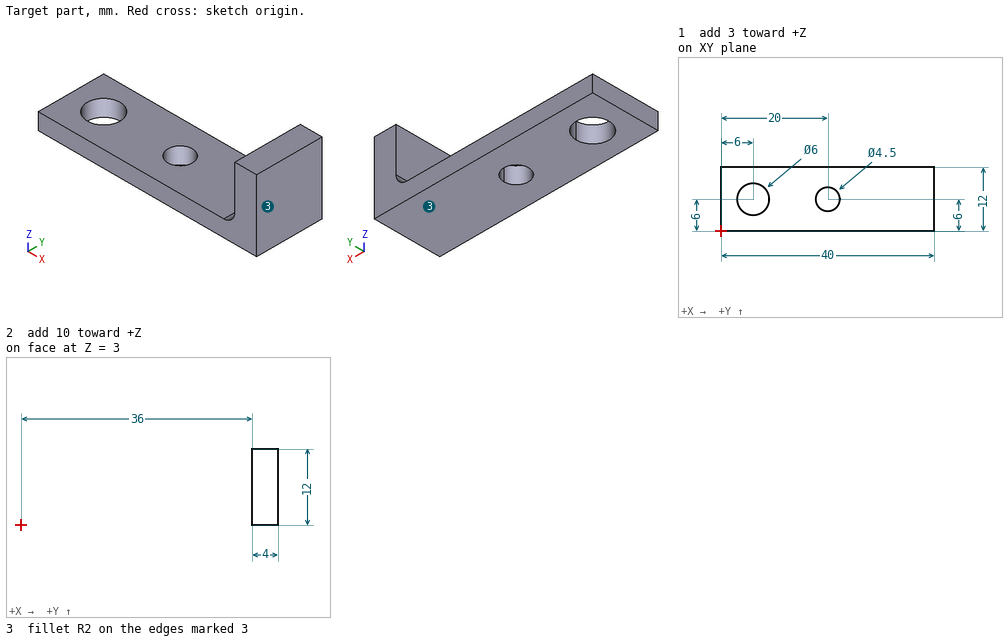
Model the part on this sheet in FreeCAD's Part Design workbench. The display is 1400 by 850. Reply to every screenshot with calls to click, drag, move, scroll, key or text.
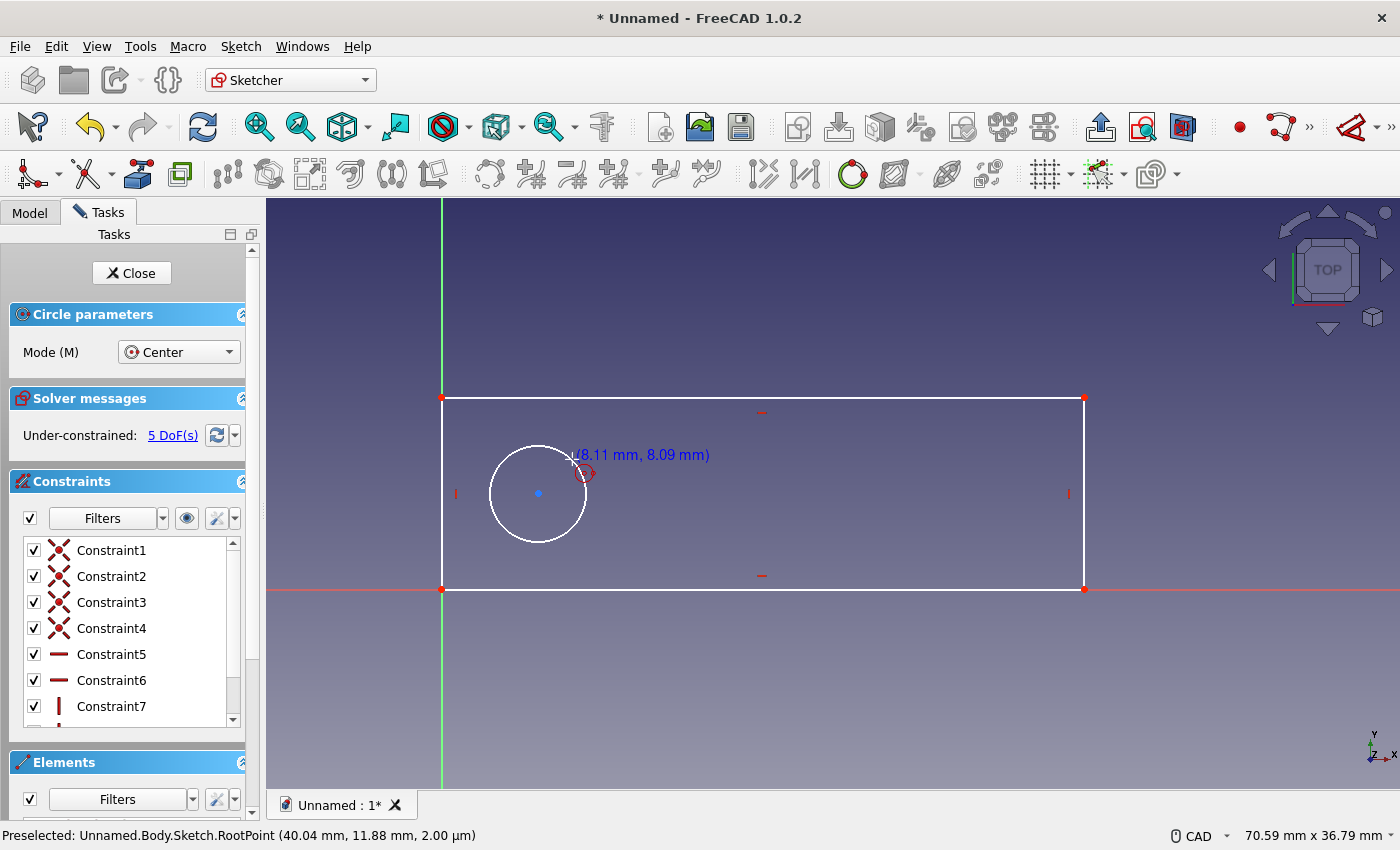
click(763, 493)
click(789, 468)
key(Escape)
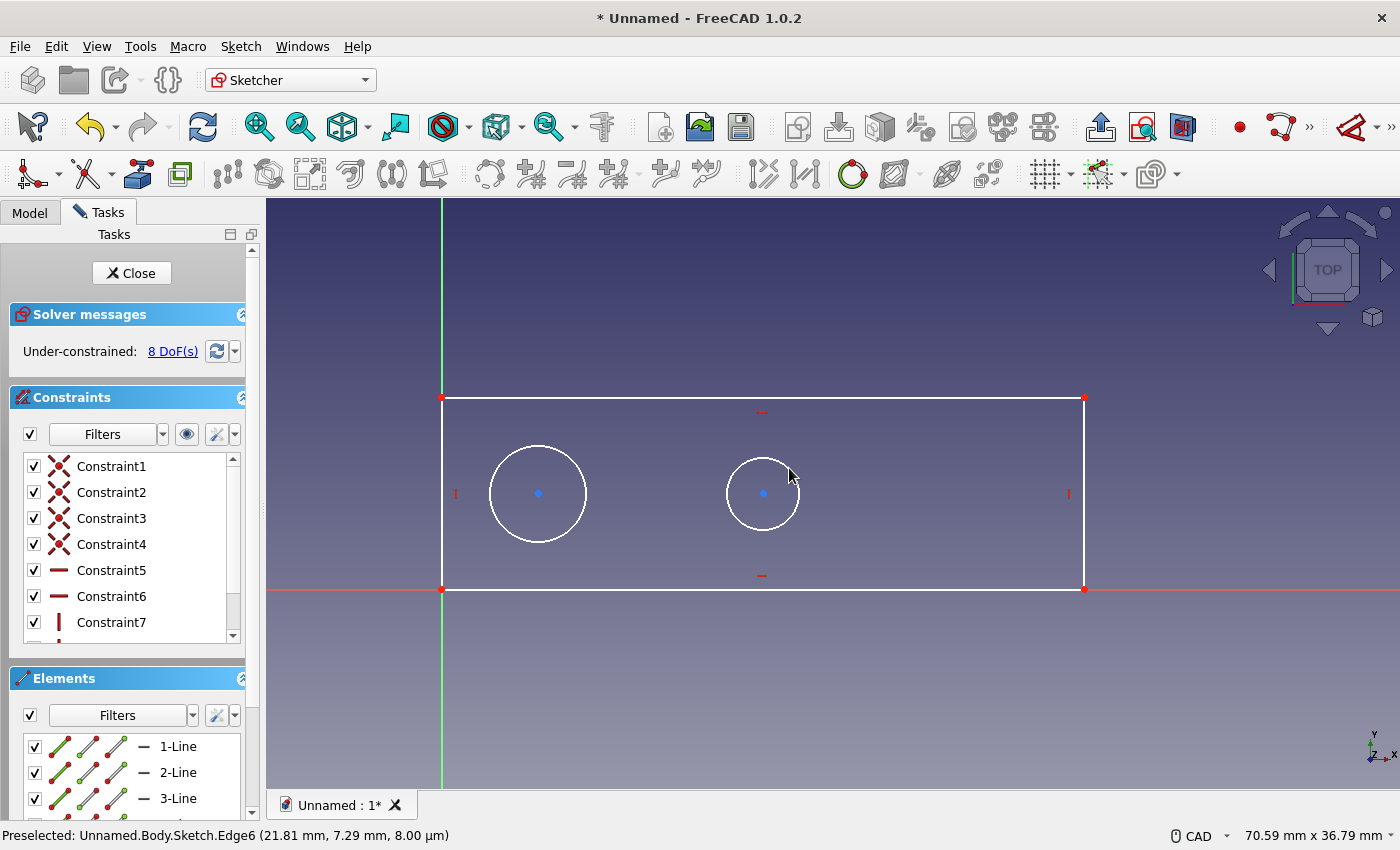
click(572, 460)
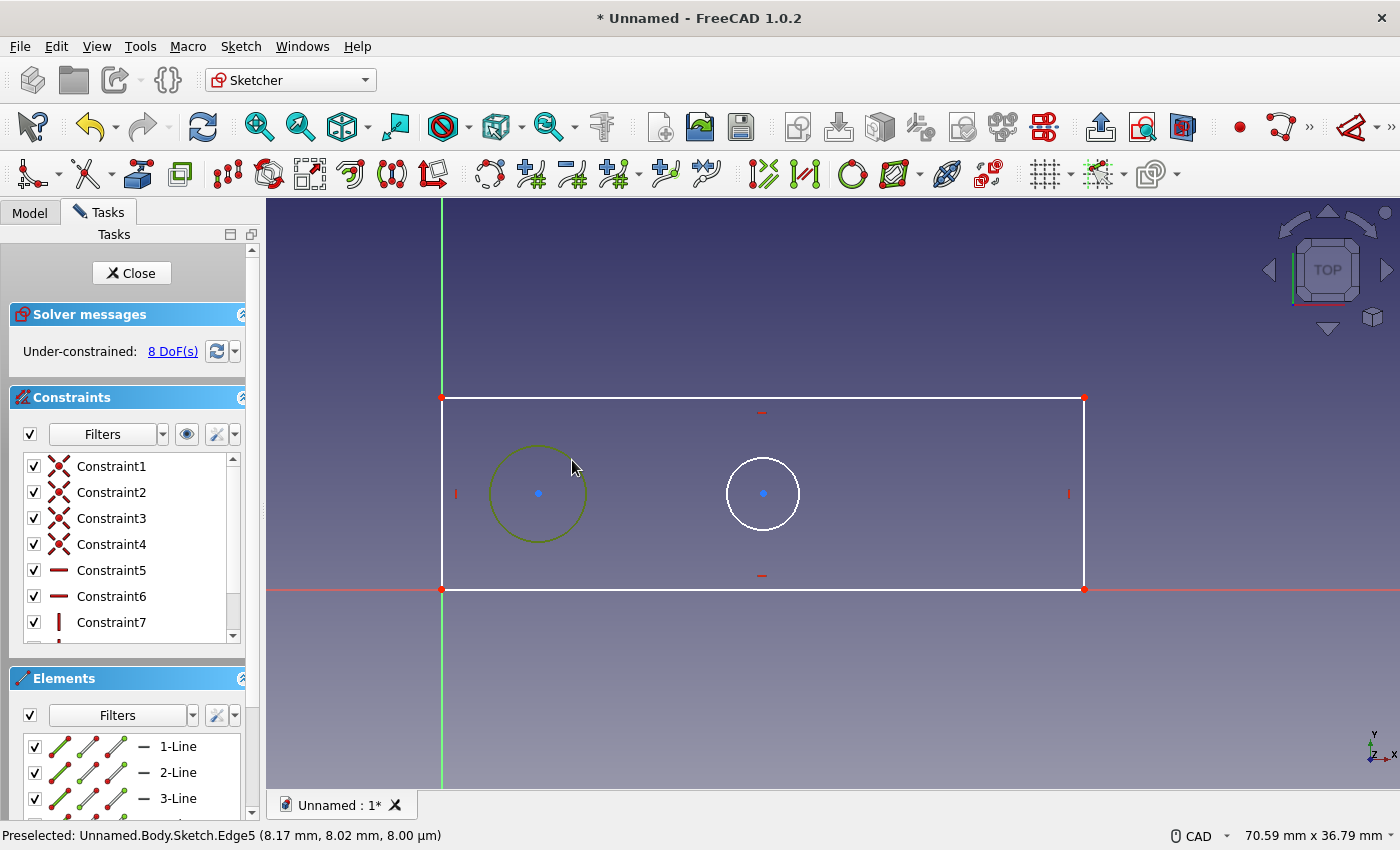
key(k)
key(o)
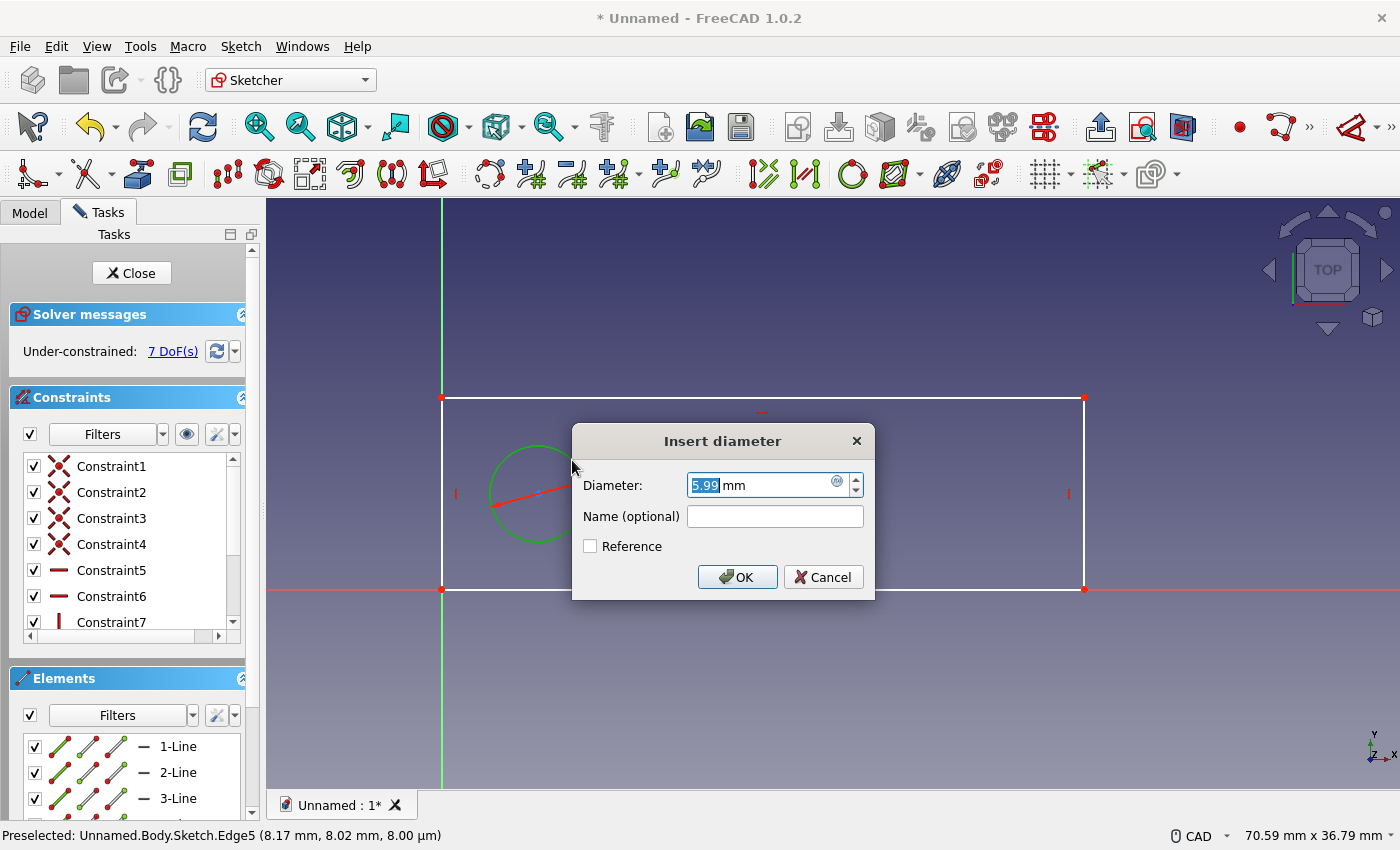
text(6)
key(Return)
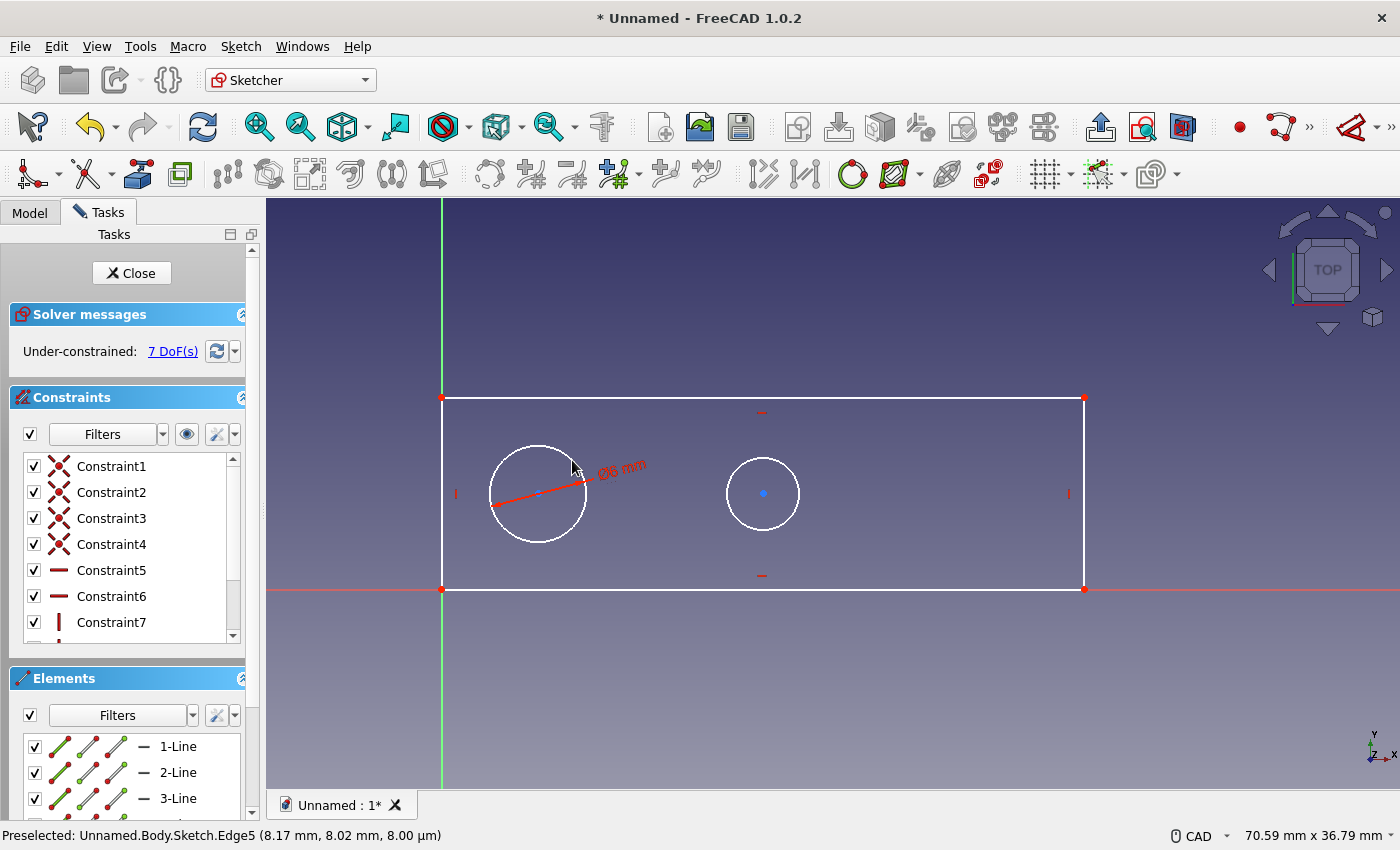
click(788, 468)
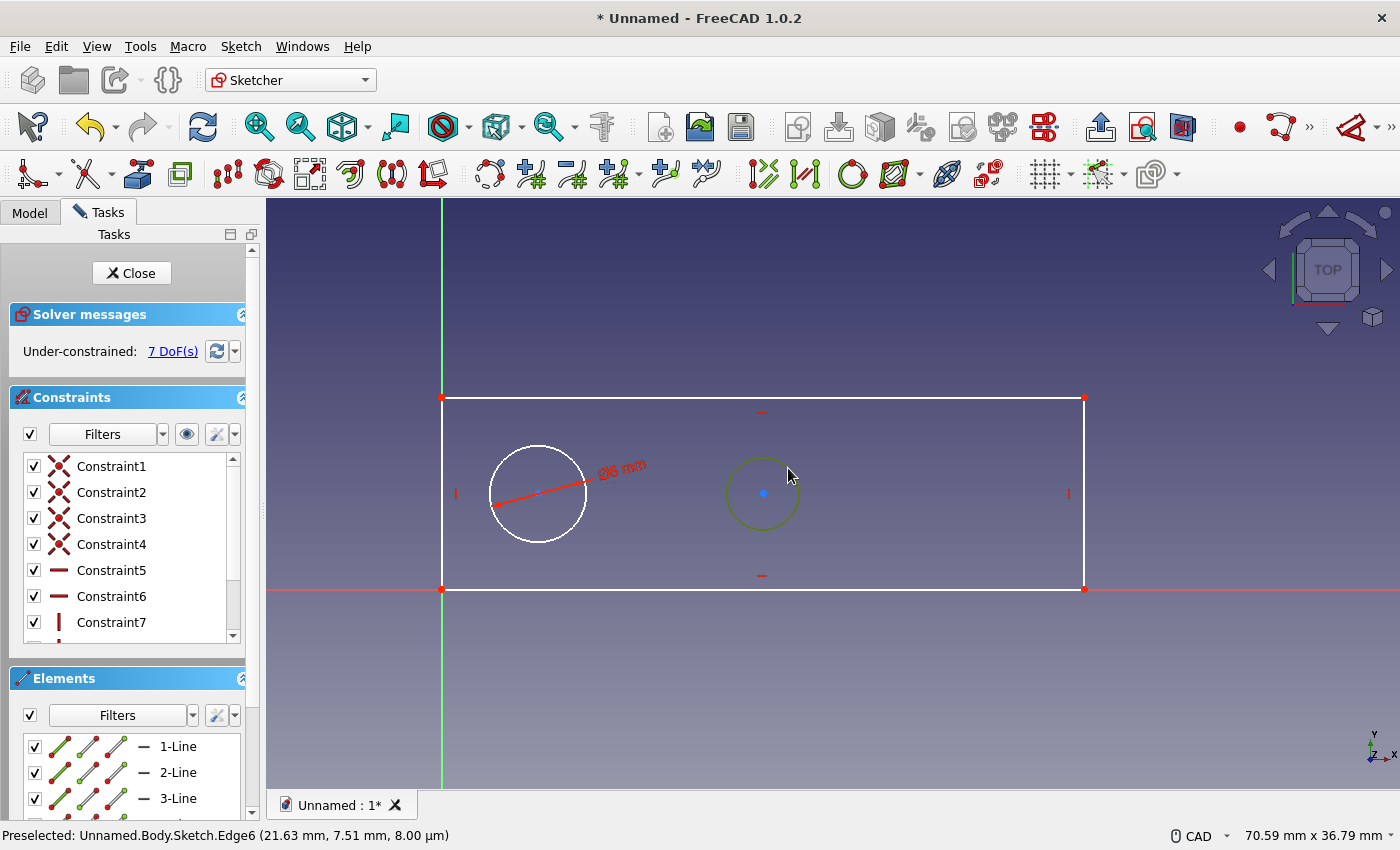
key(k)
key(o)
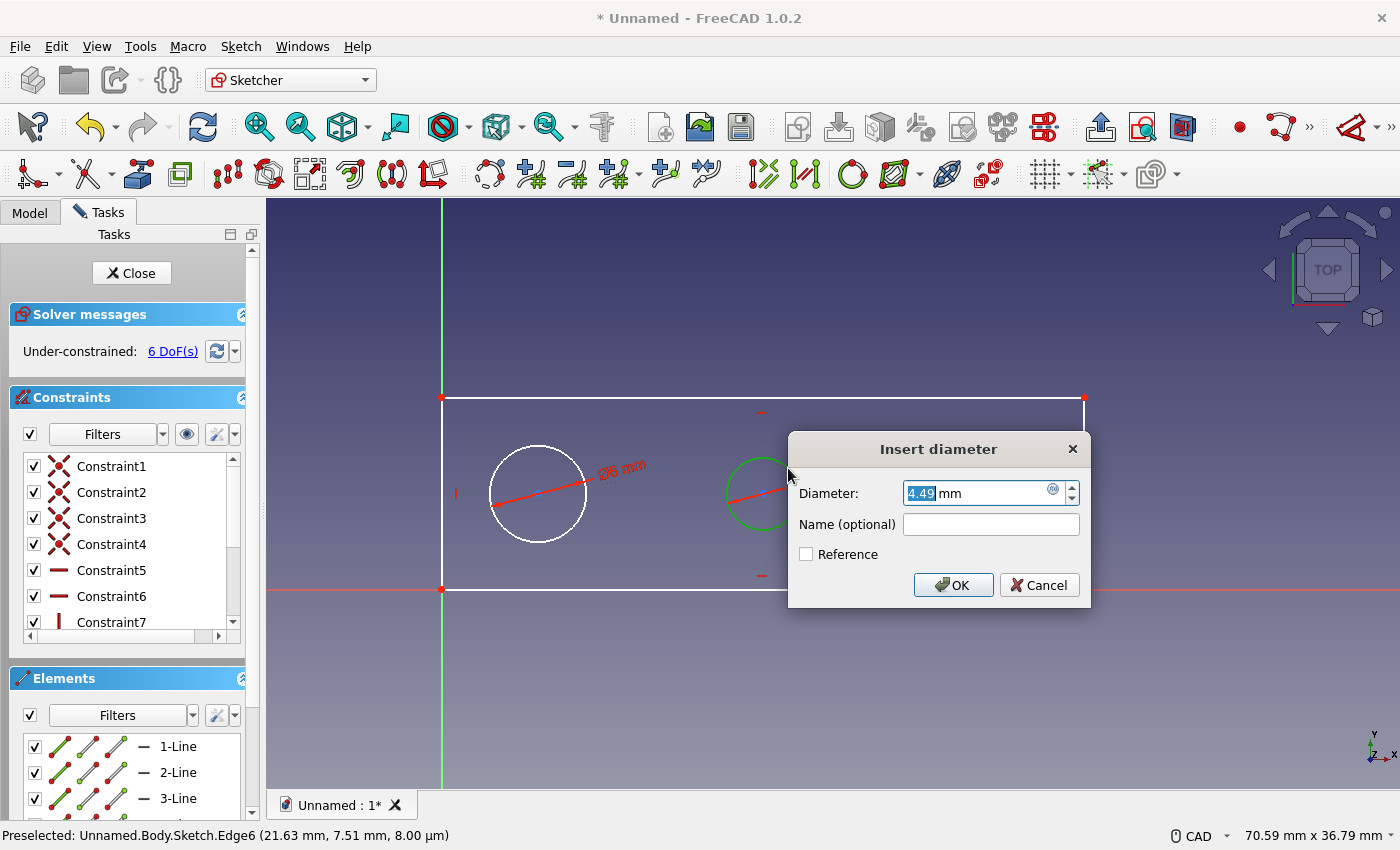
text(4.5)
key(Return)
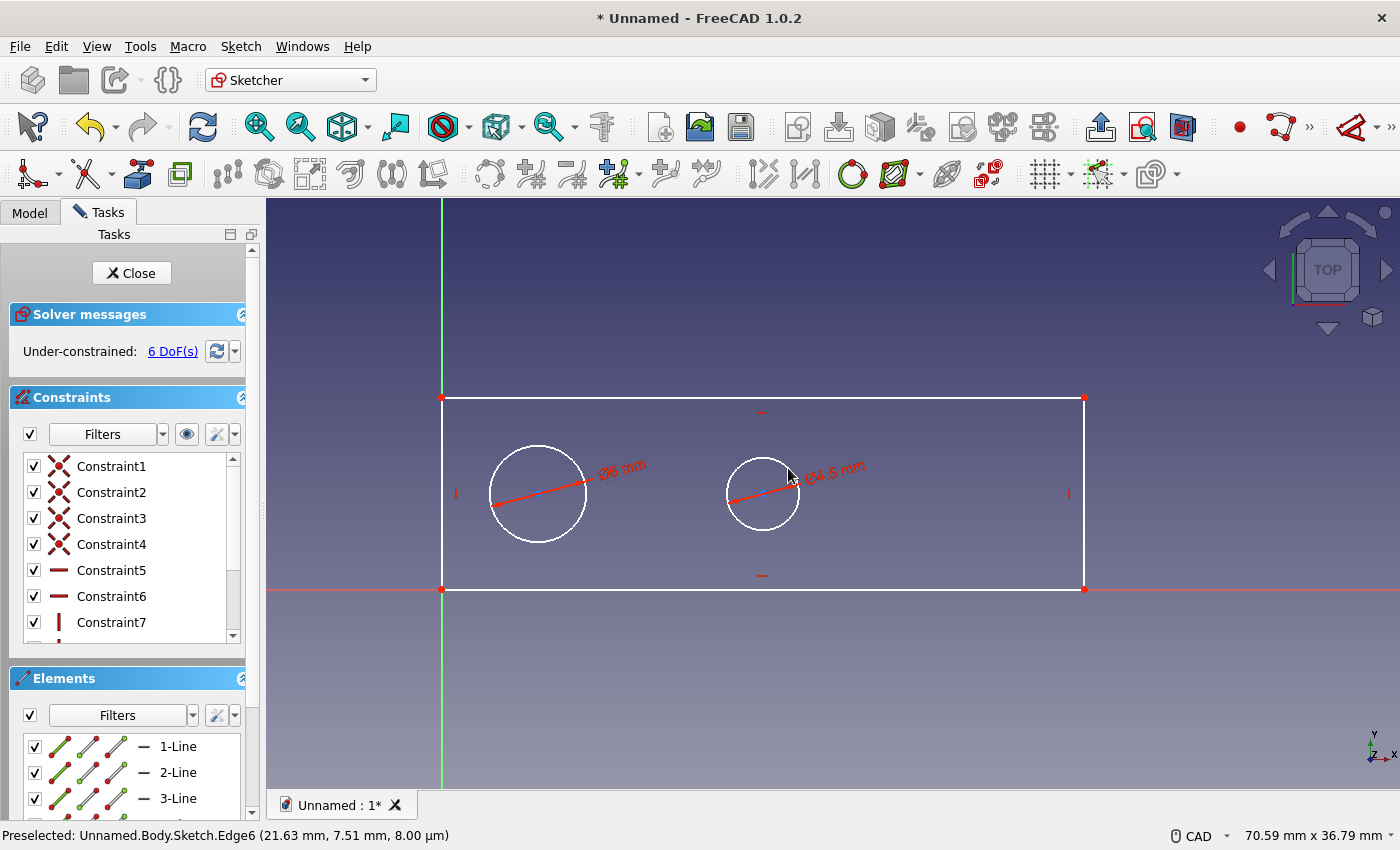
click(538, 494)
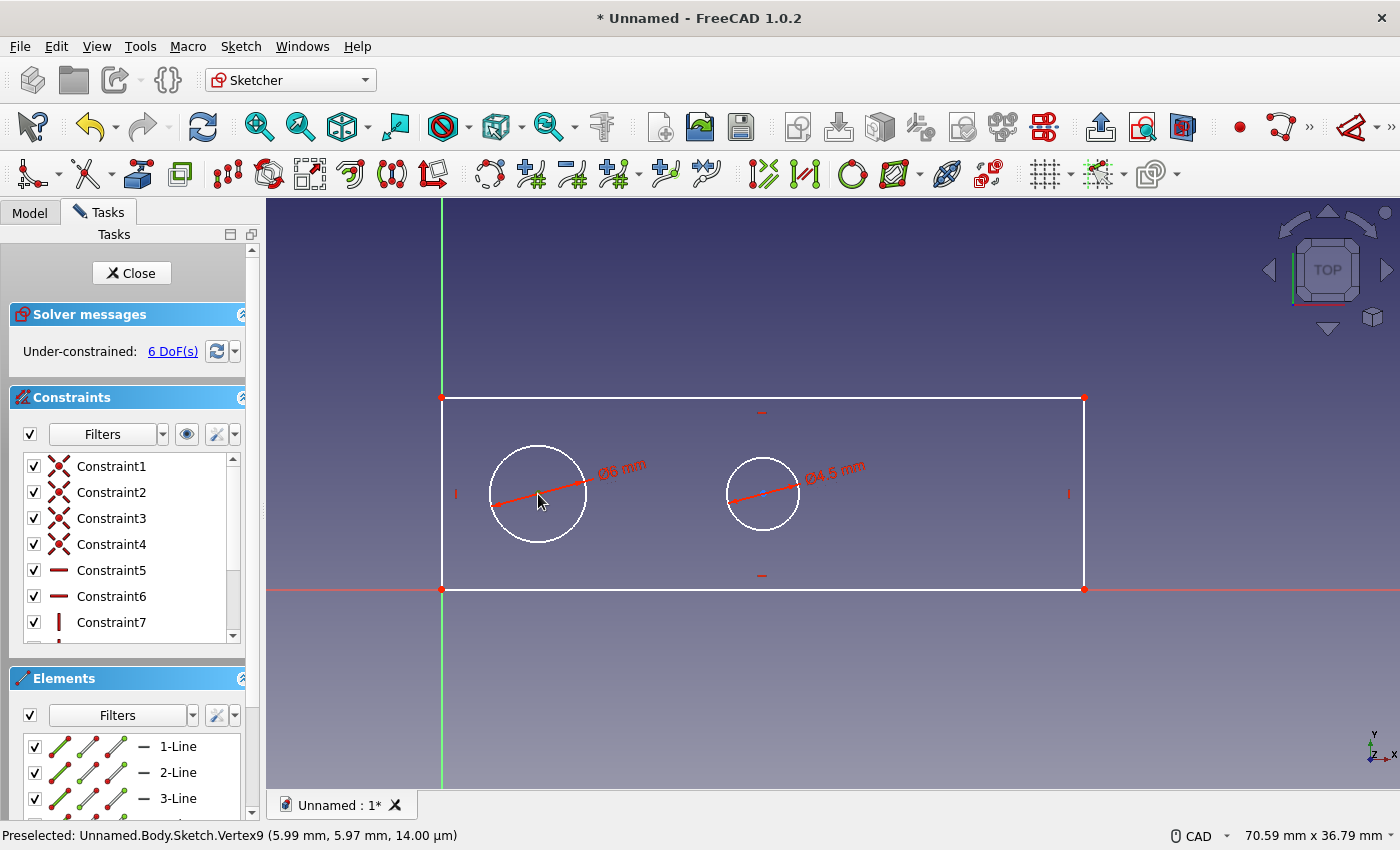
key(l)